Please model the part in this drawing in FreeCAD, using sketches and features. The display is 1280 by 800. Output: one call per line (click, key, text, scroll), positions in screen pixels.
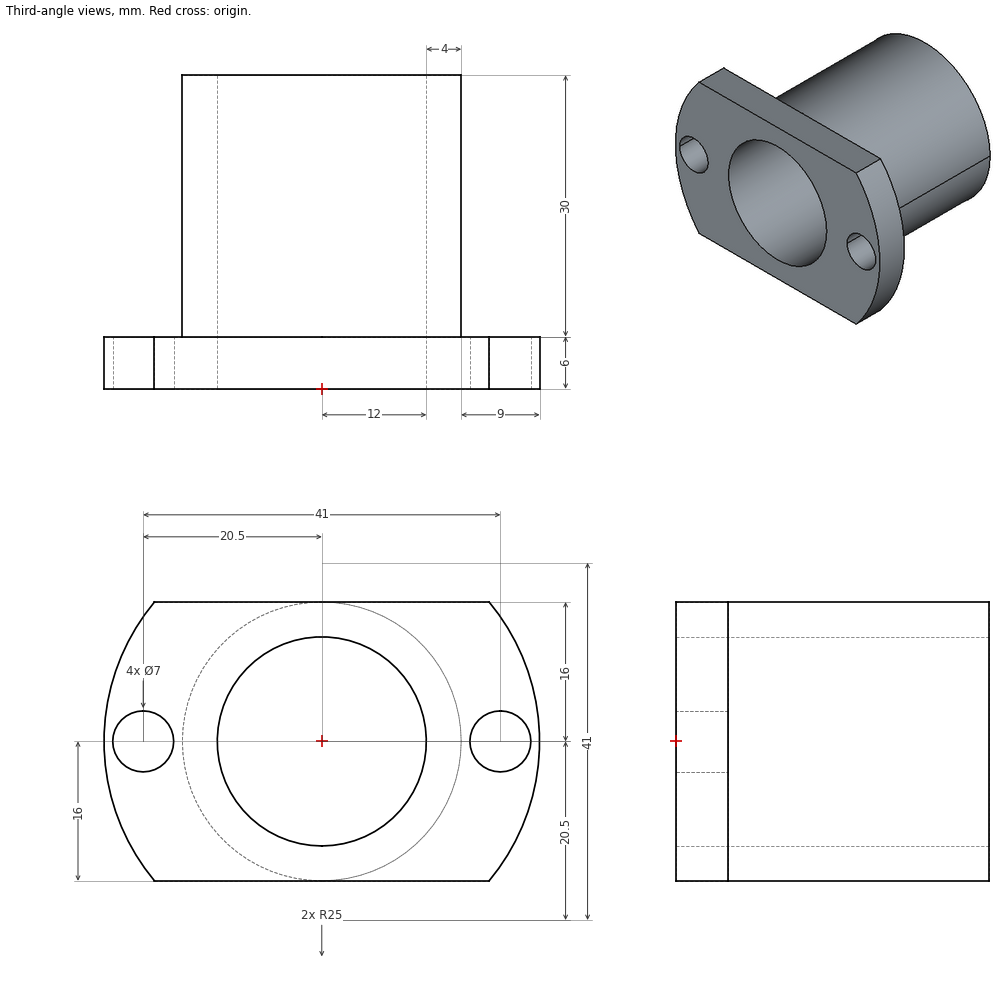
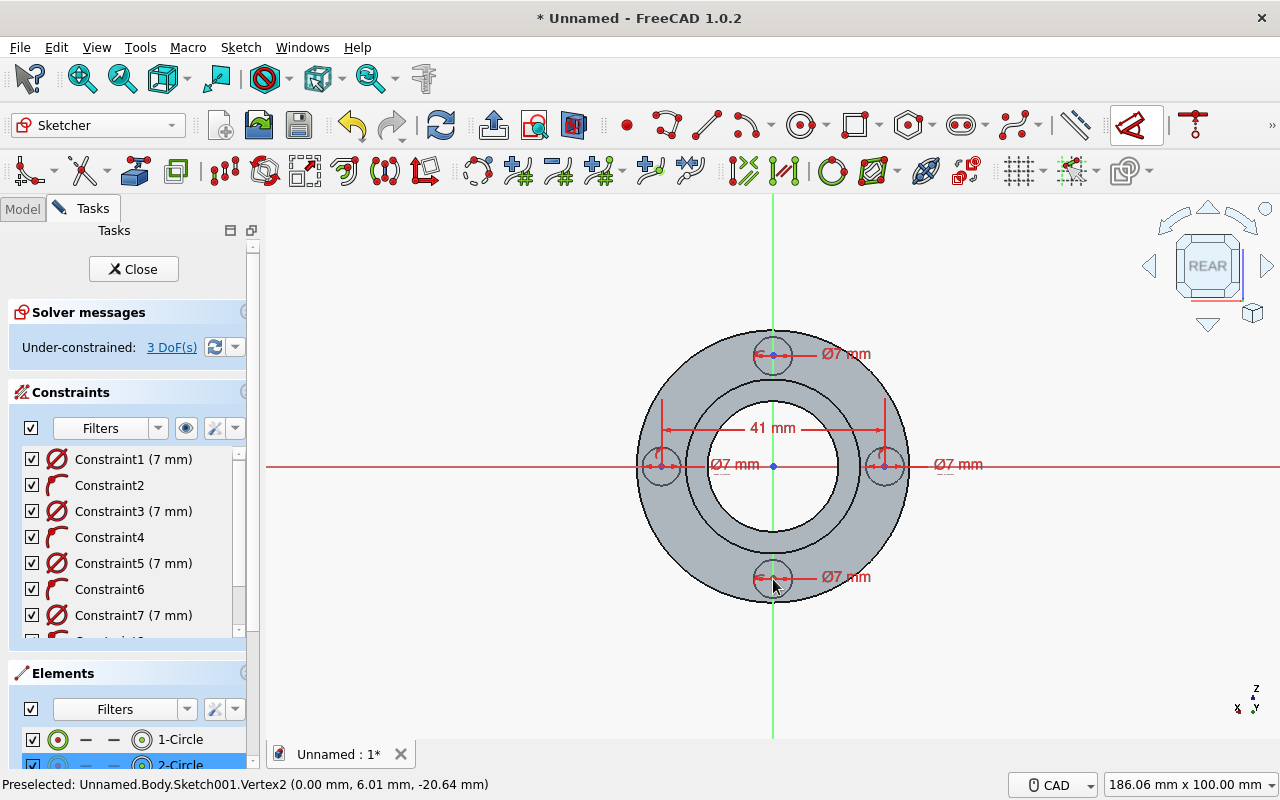
click(773, 356)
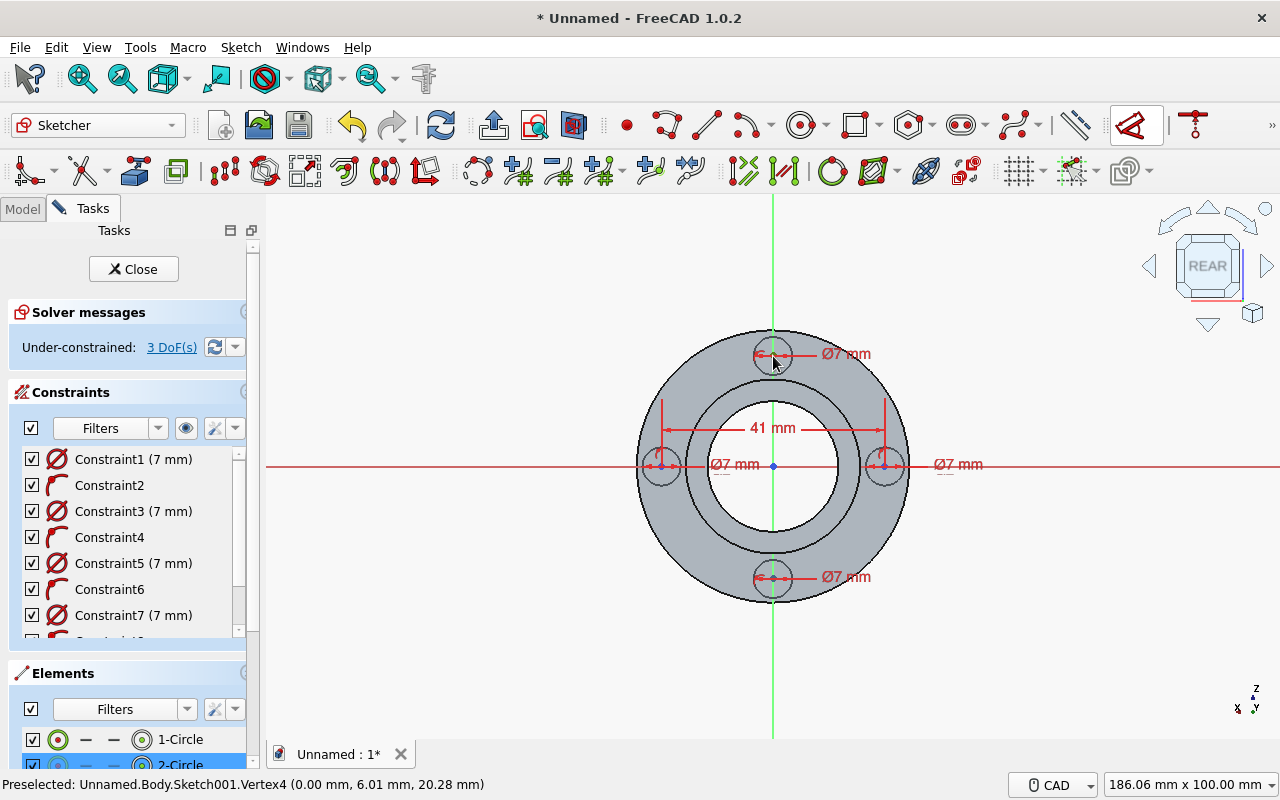
click(1158, 126)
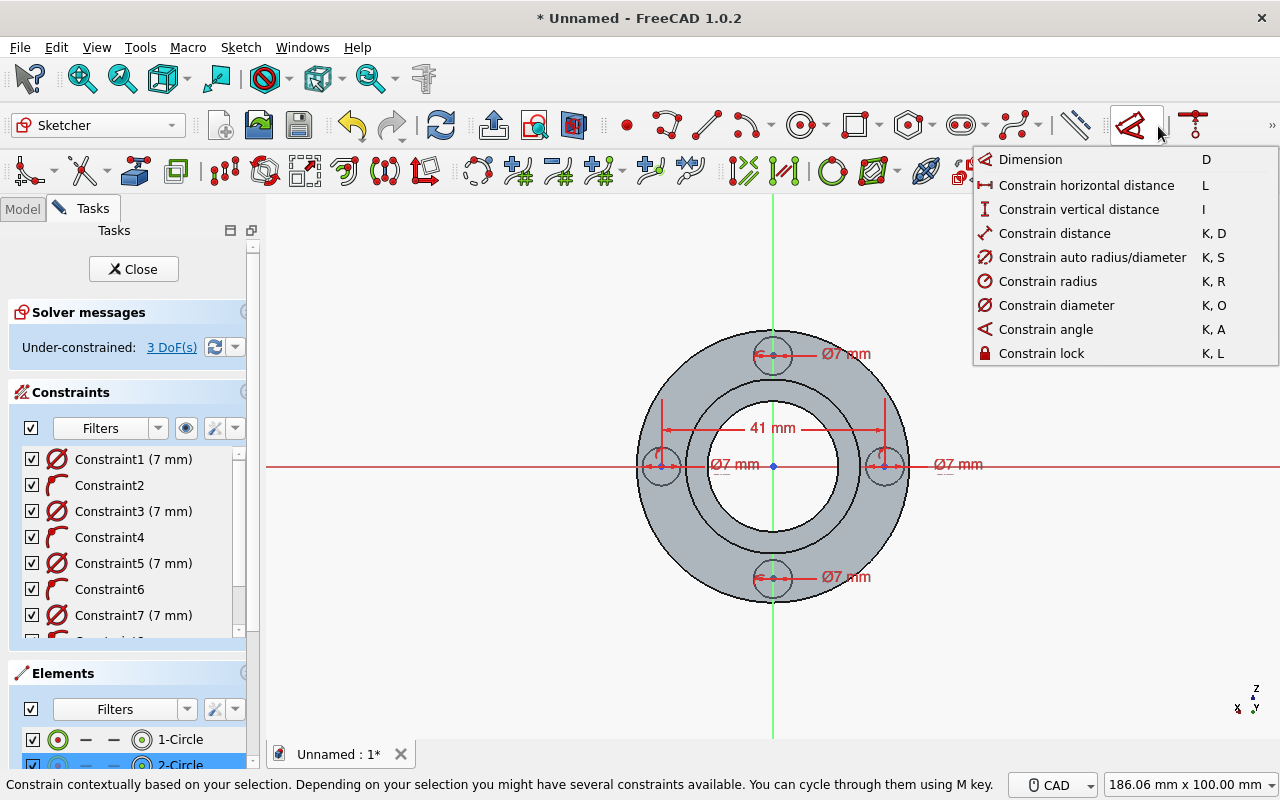
click(1126, 209)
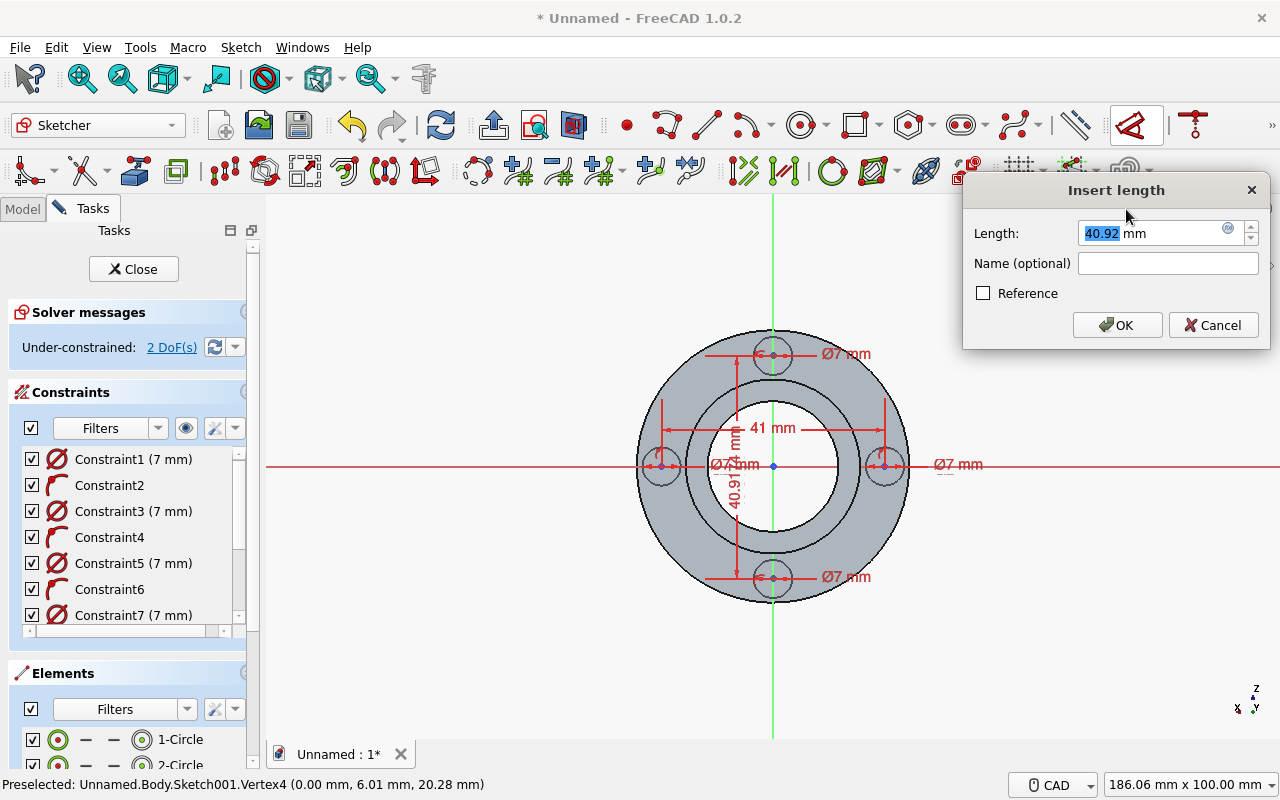
text(41)
key(Return)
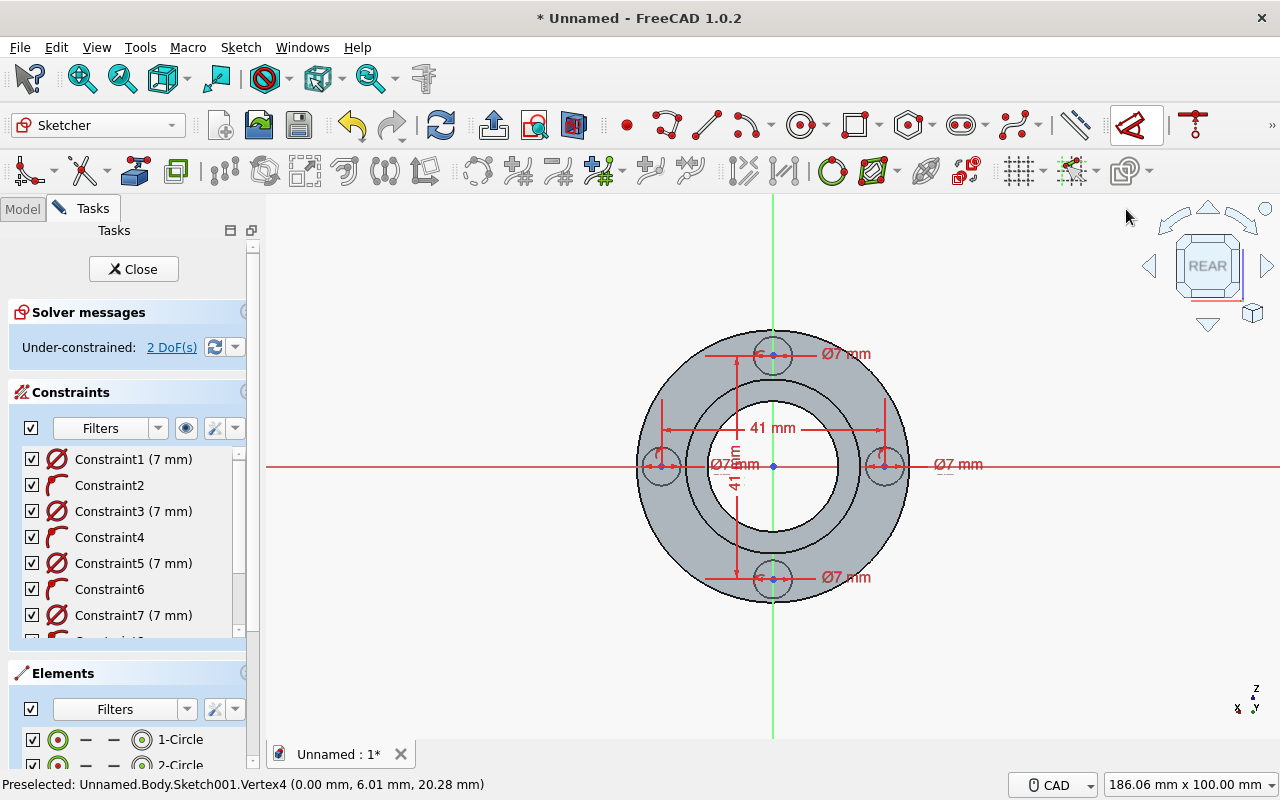
click(885, 466)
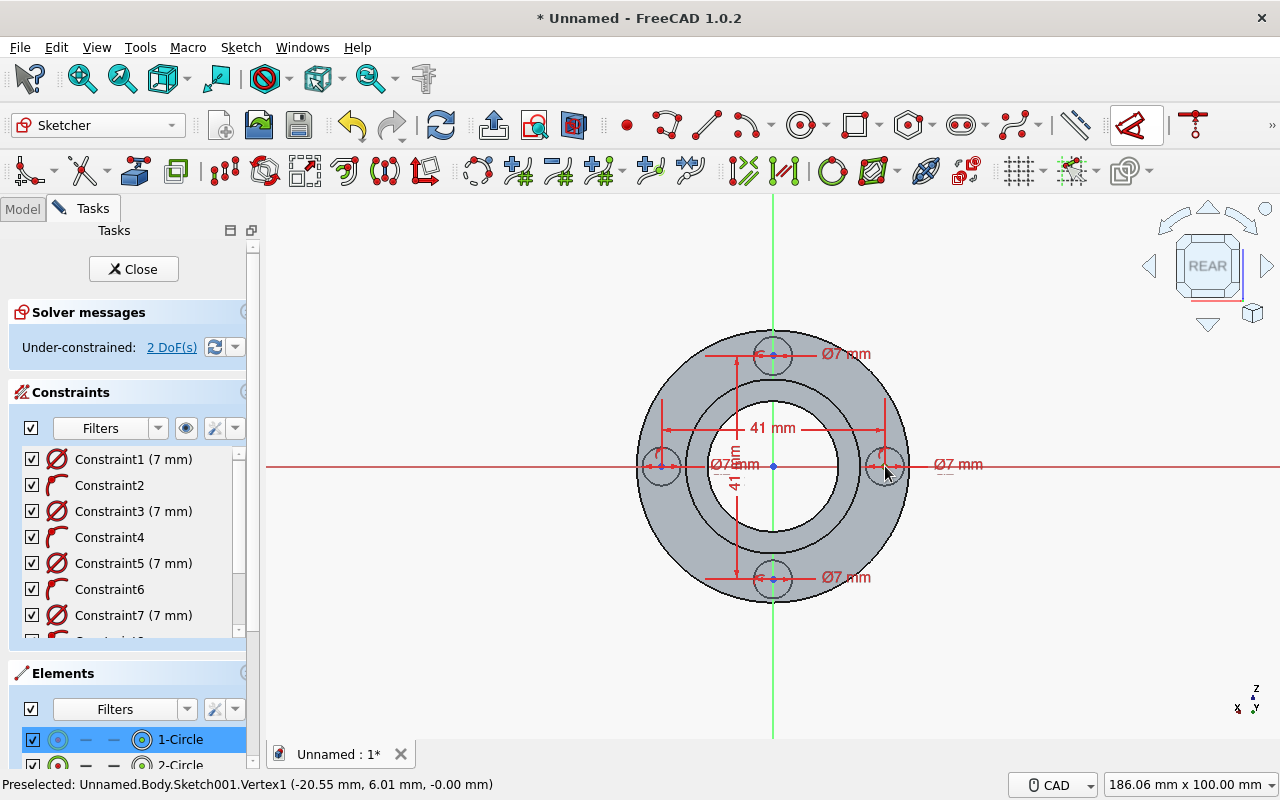
click(1158, 126)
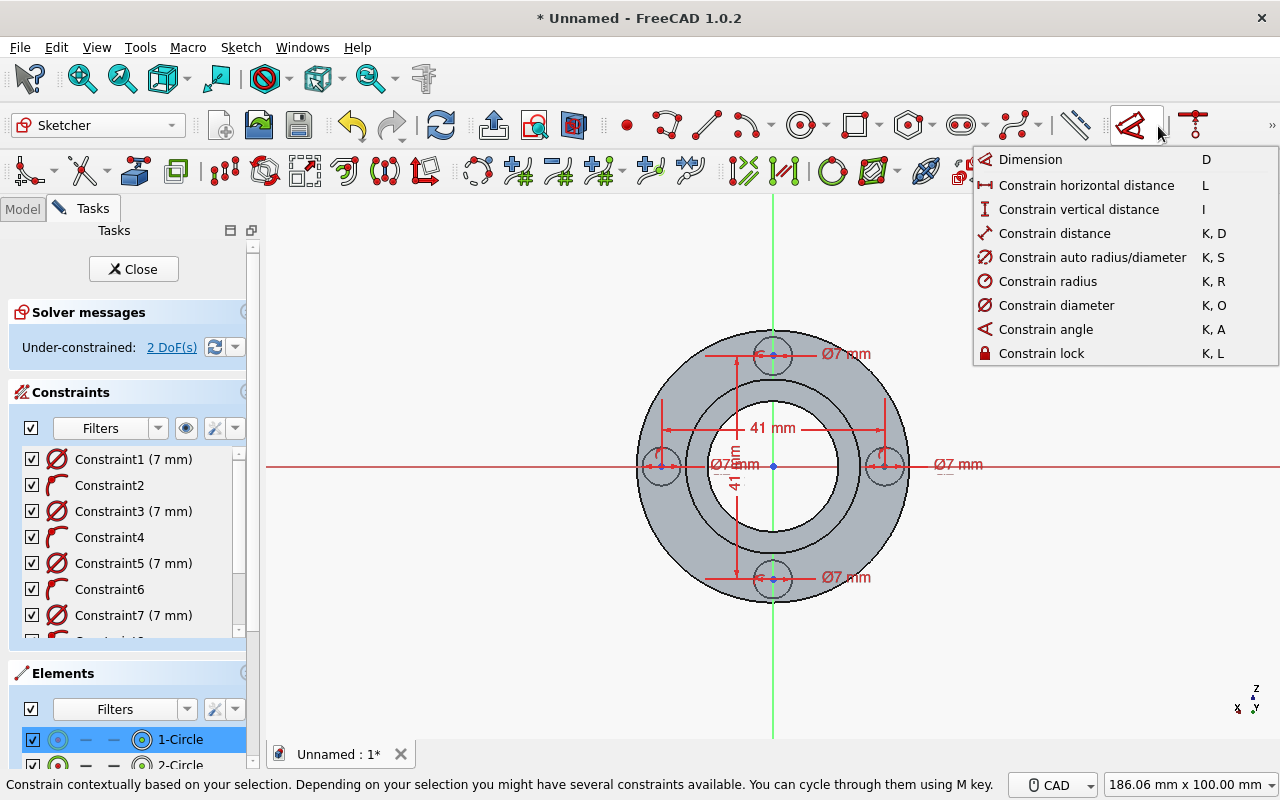
click(1126, 185)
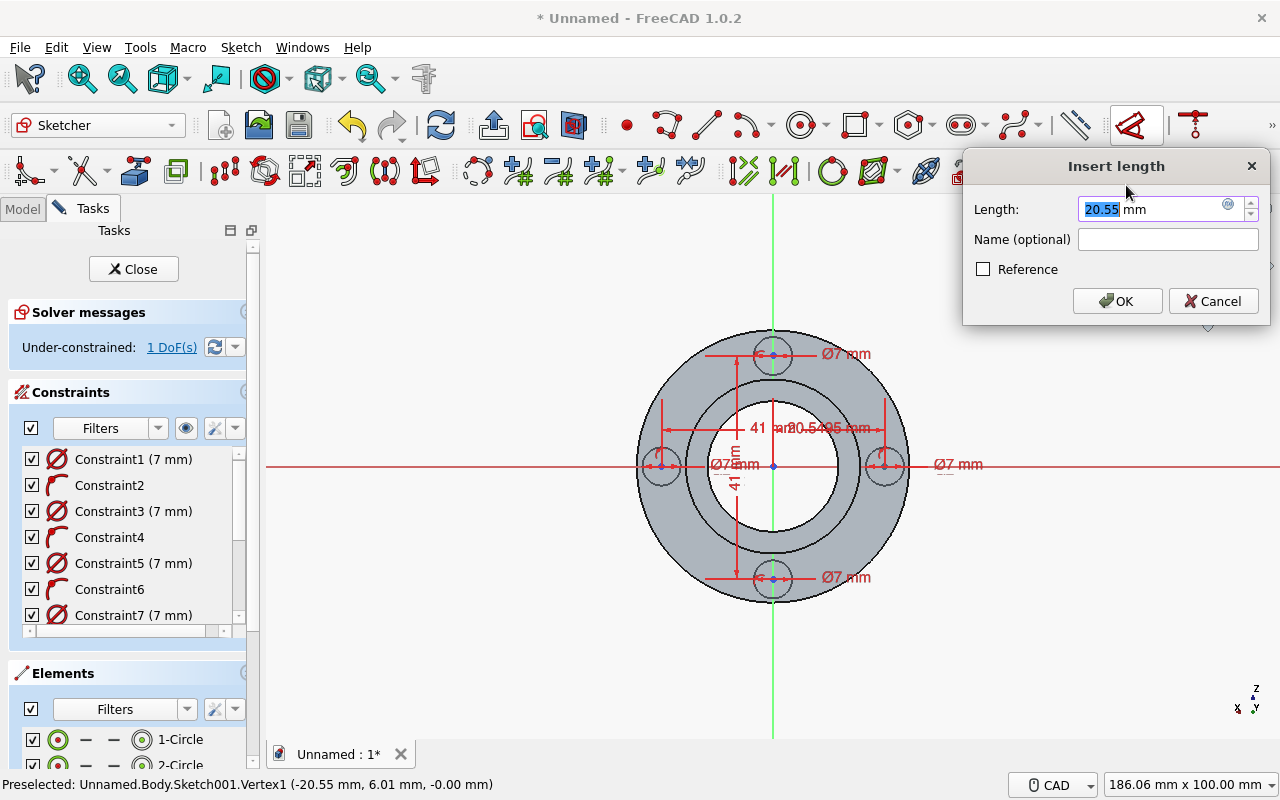
text(20.5)
key(Return)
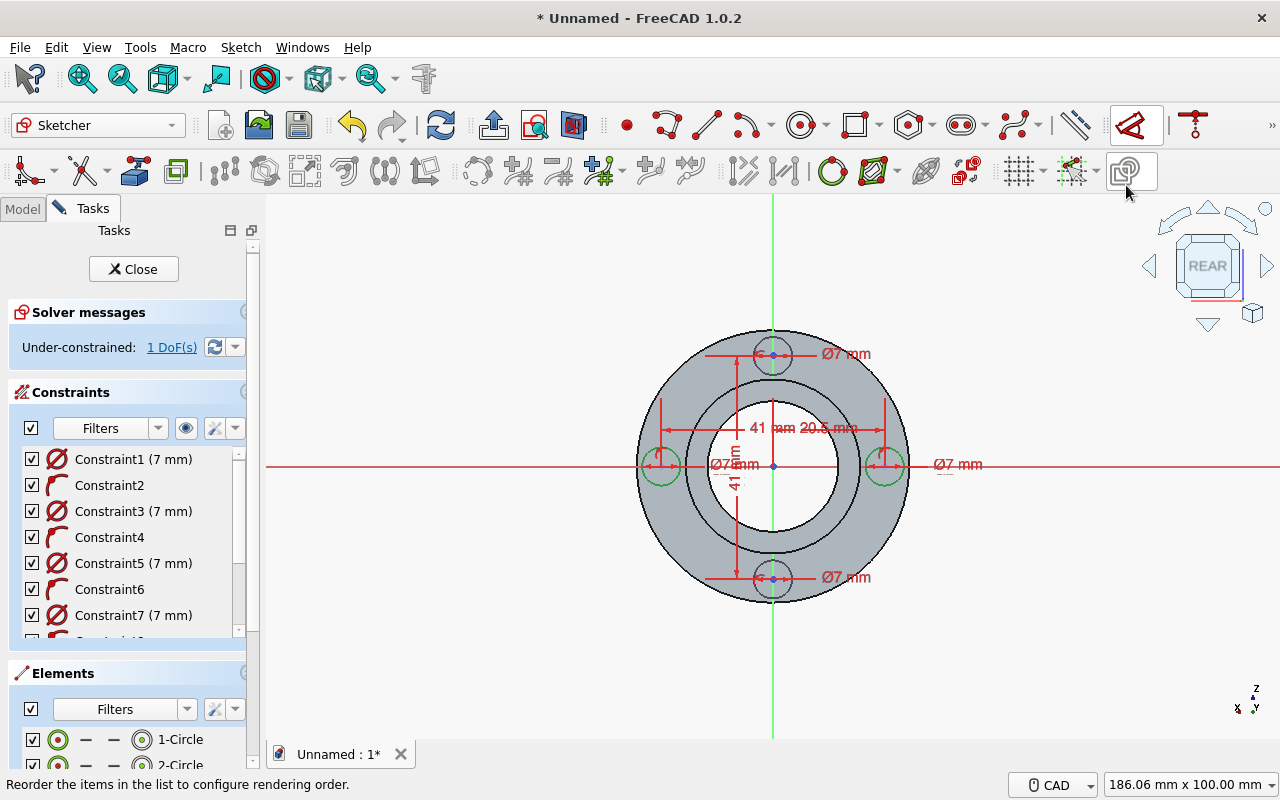
click(773, 579)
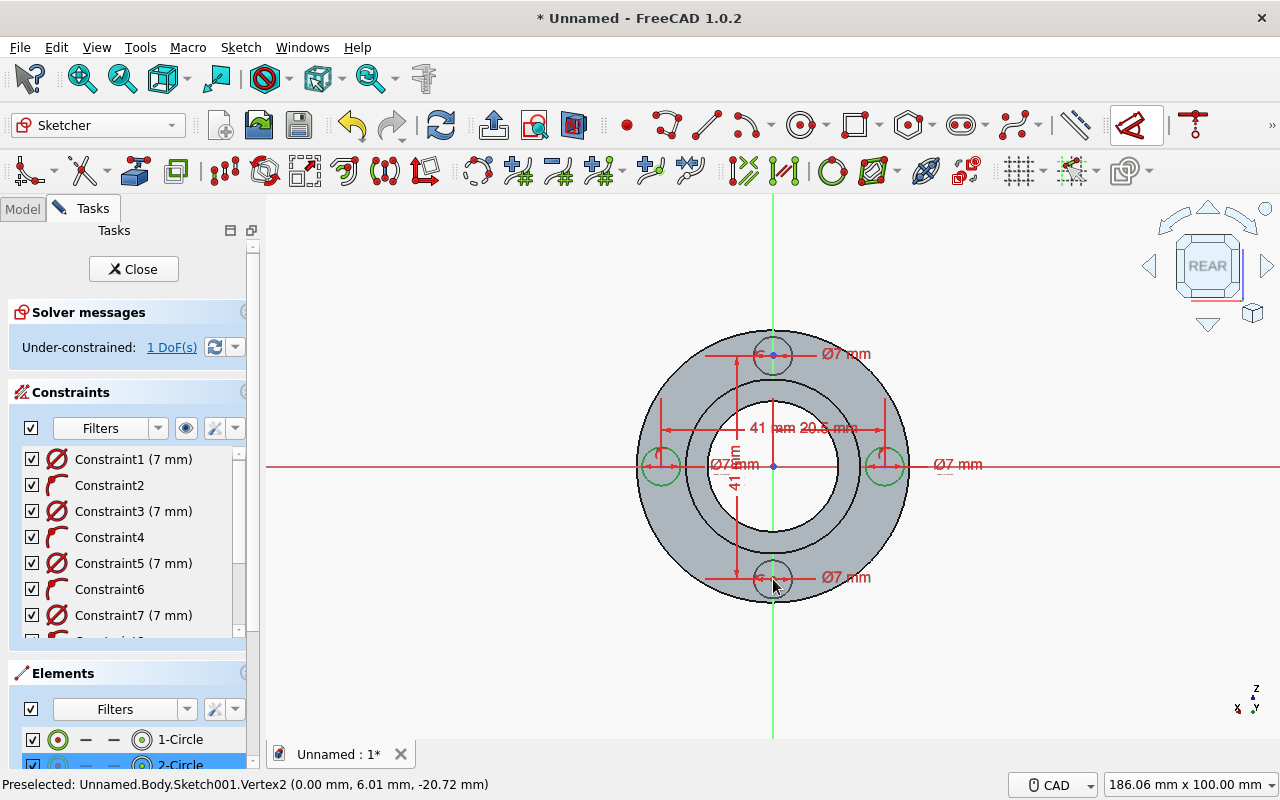
click(1158, 126)